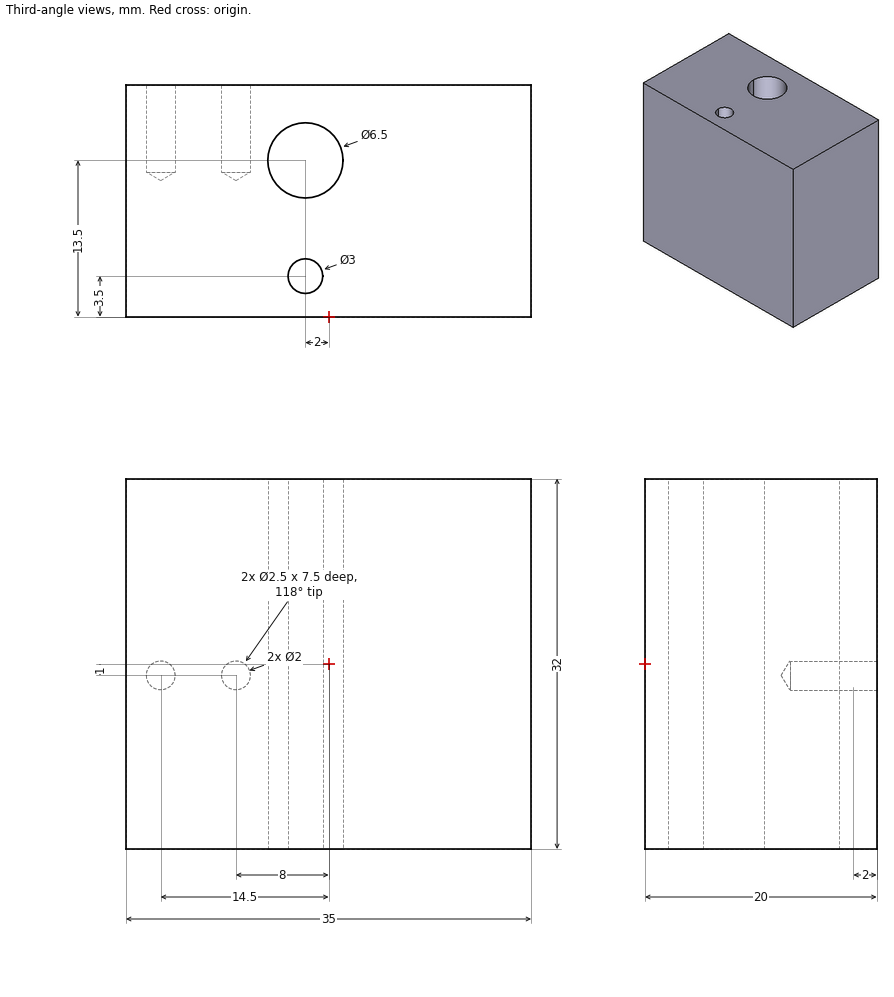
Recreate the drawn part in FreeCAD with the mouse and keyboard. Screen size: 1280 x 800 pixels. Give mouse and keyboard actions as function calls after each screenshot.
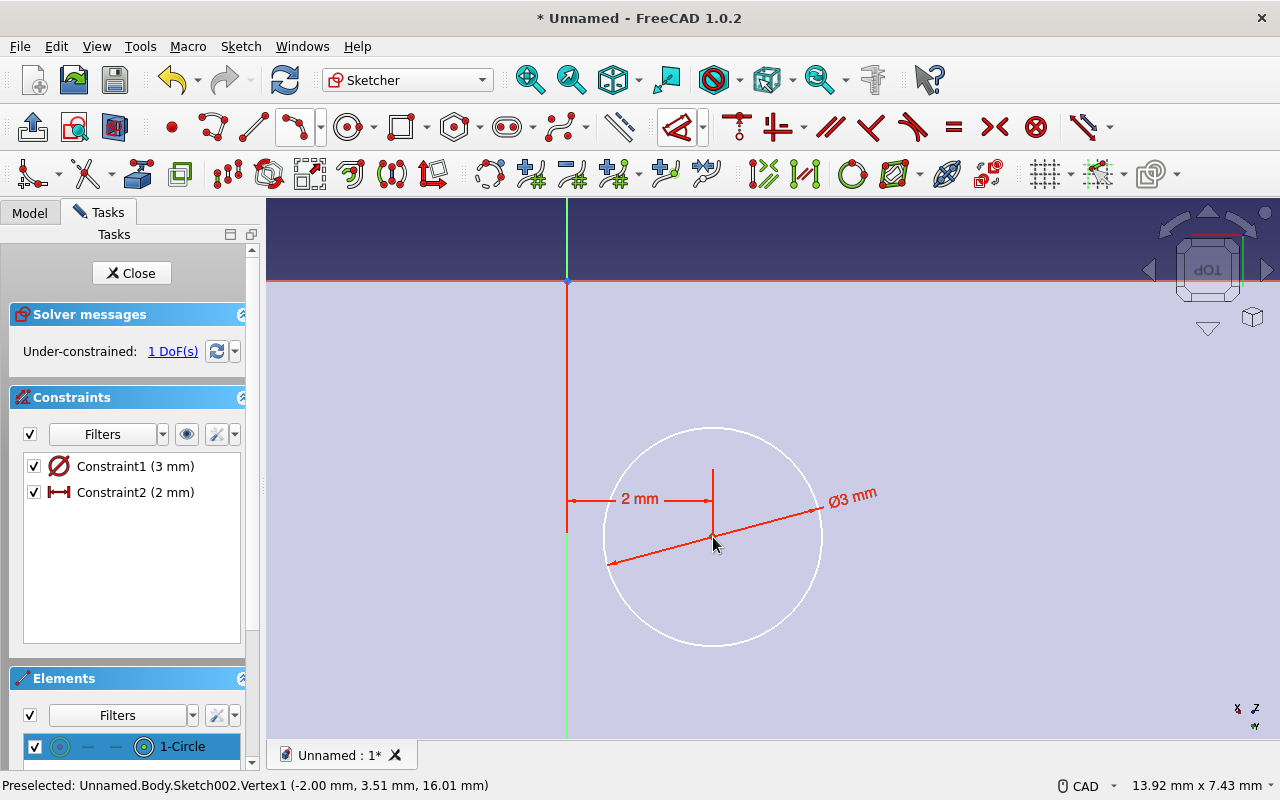
click(702, 128)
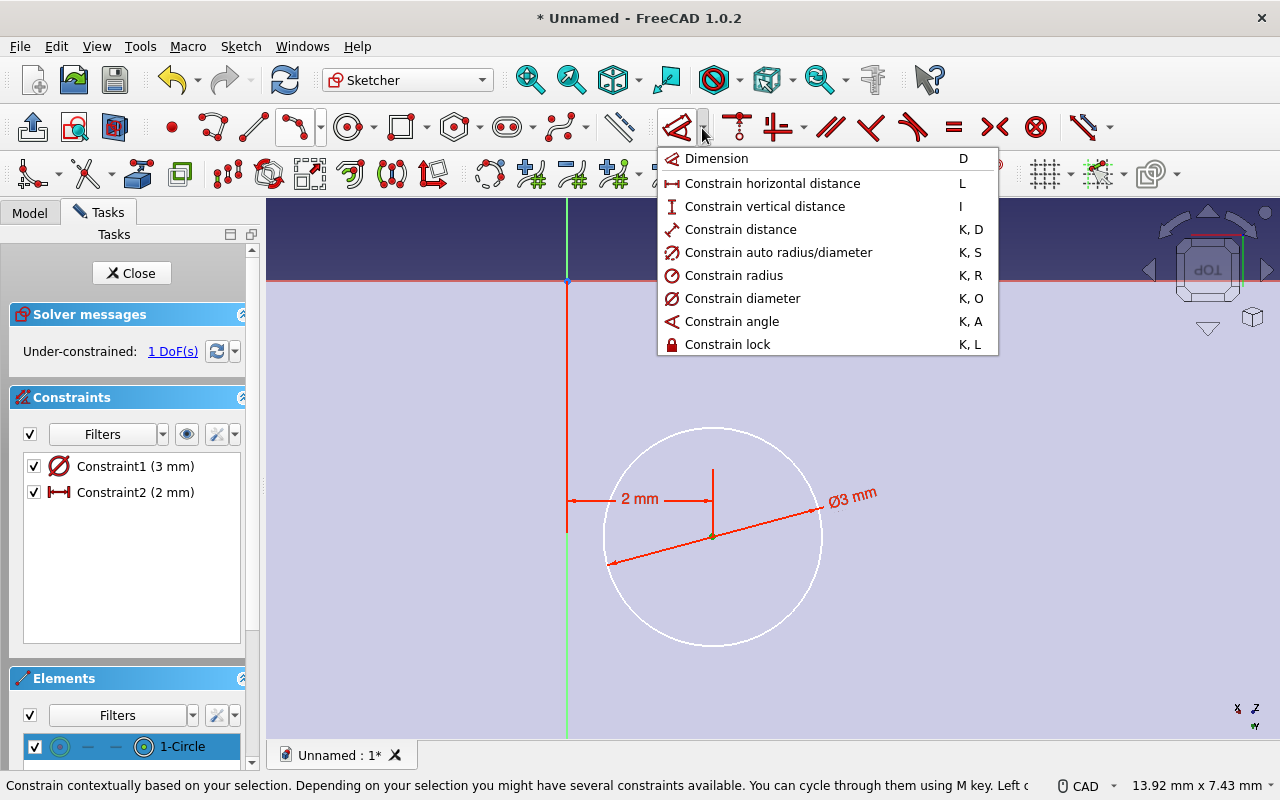
click(828, 206)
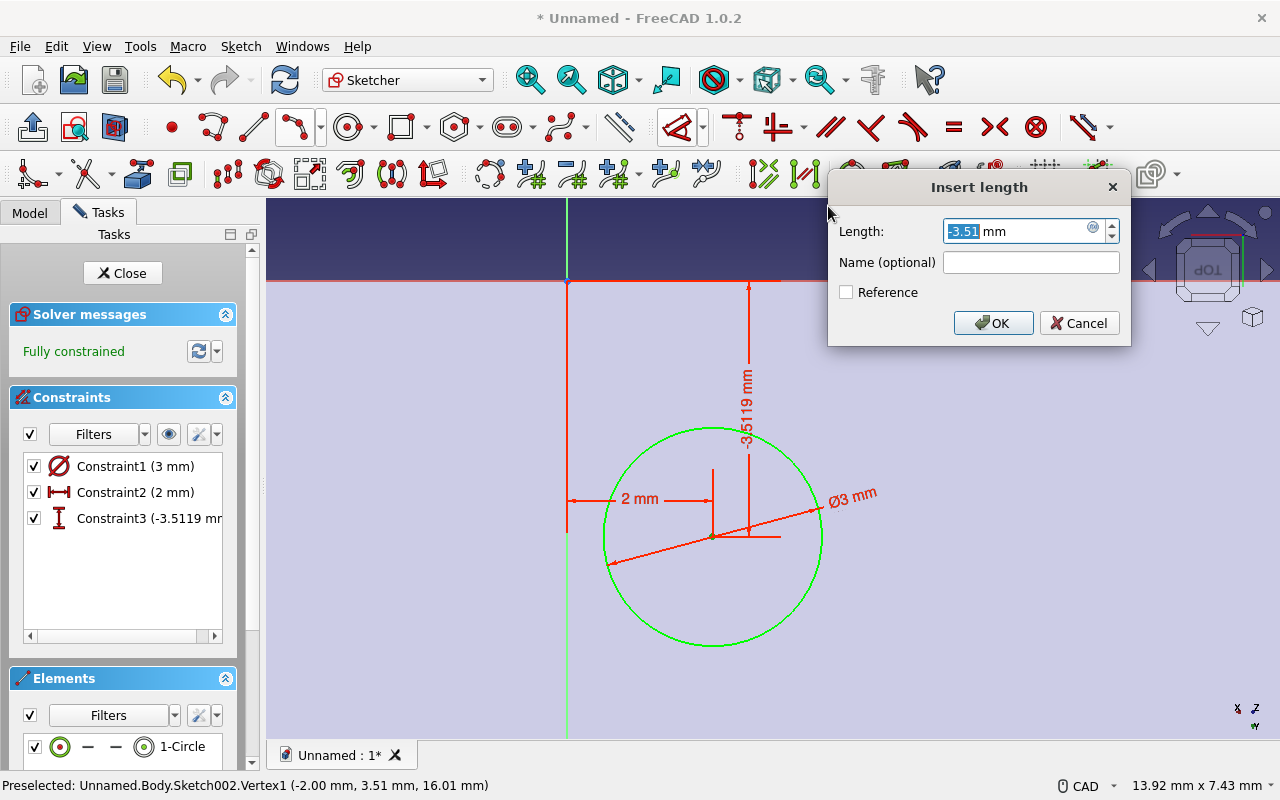
text(-3.5)
key(Return)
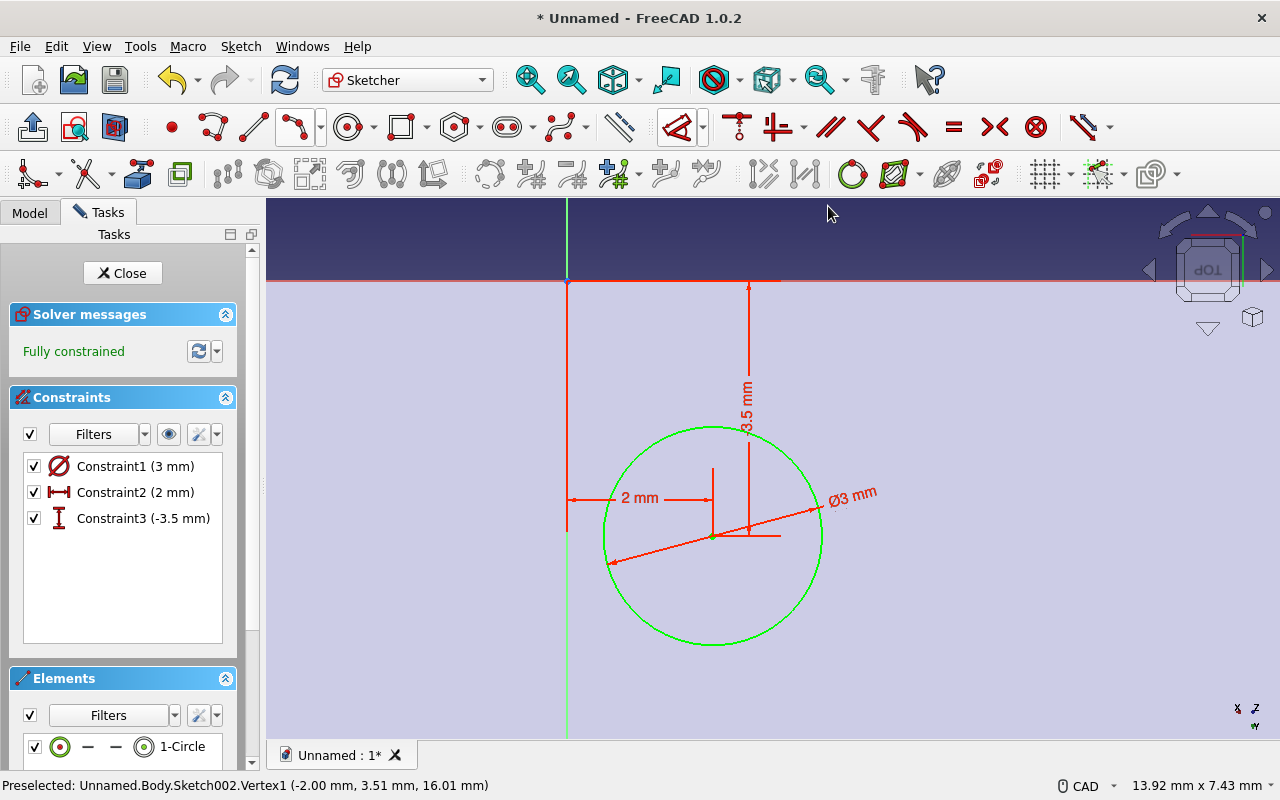
click(123, 273)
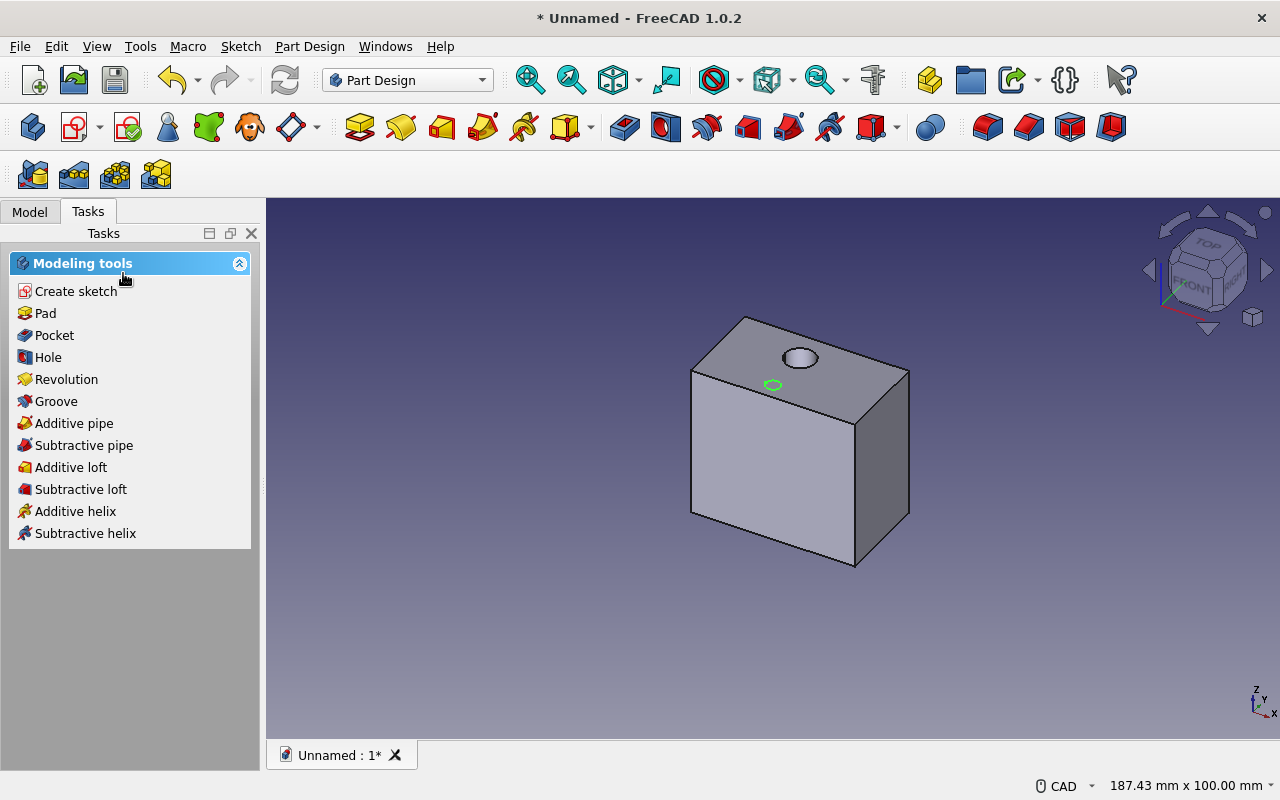
click(625, 128)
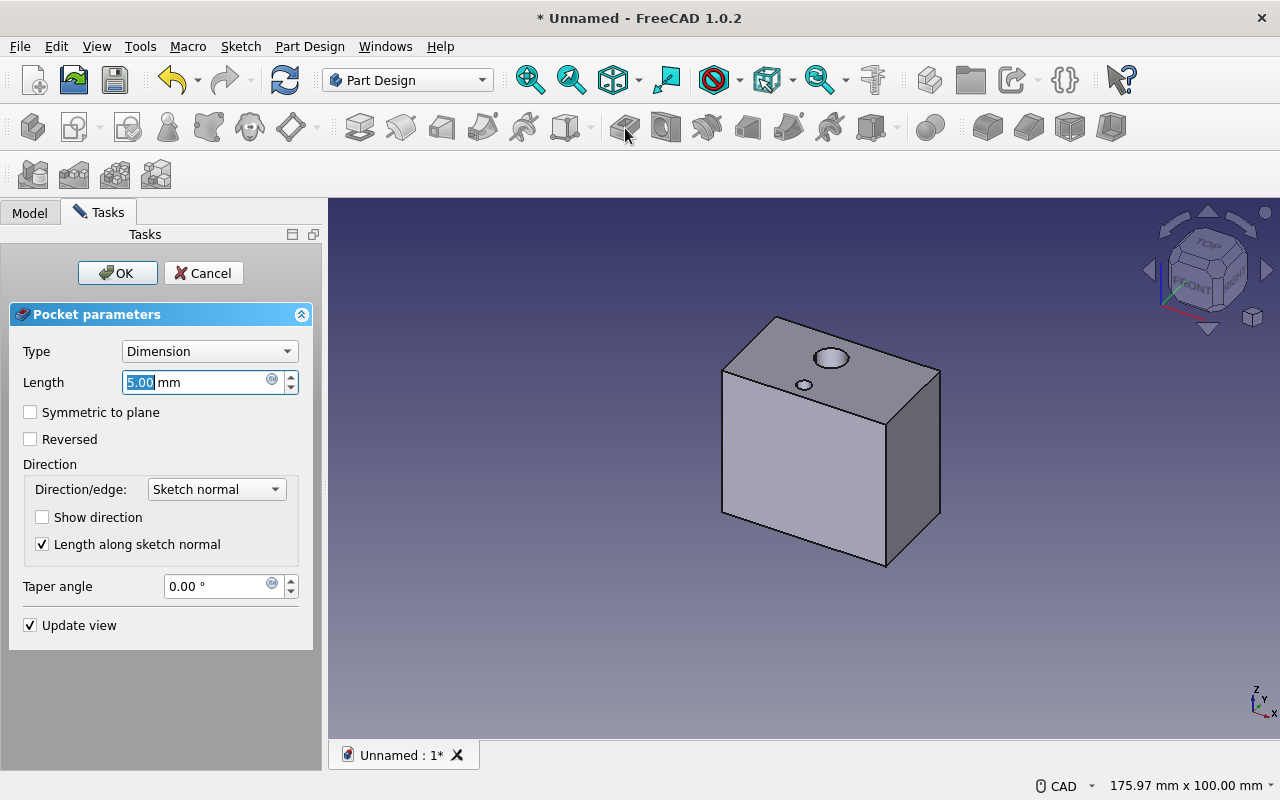
click(210, 352)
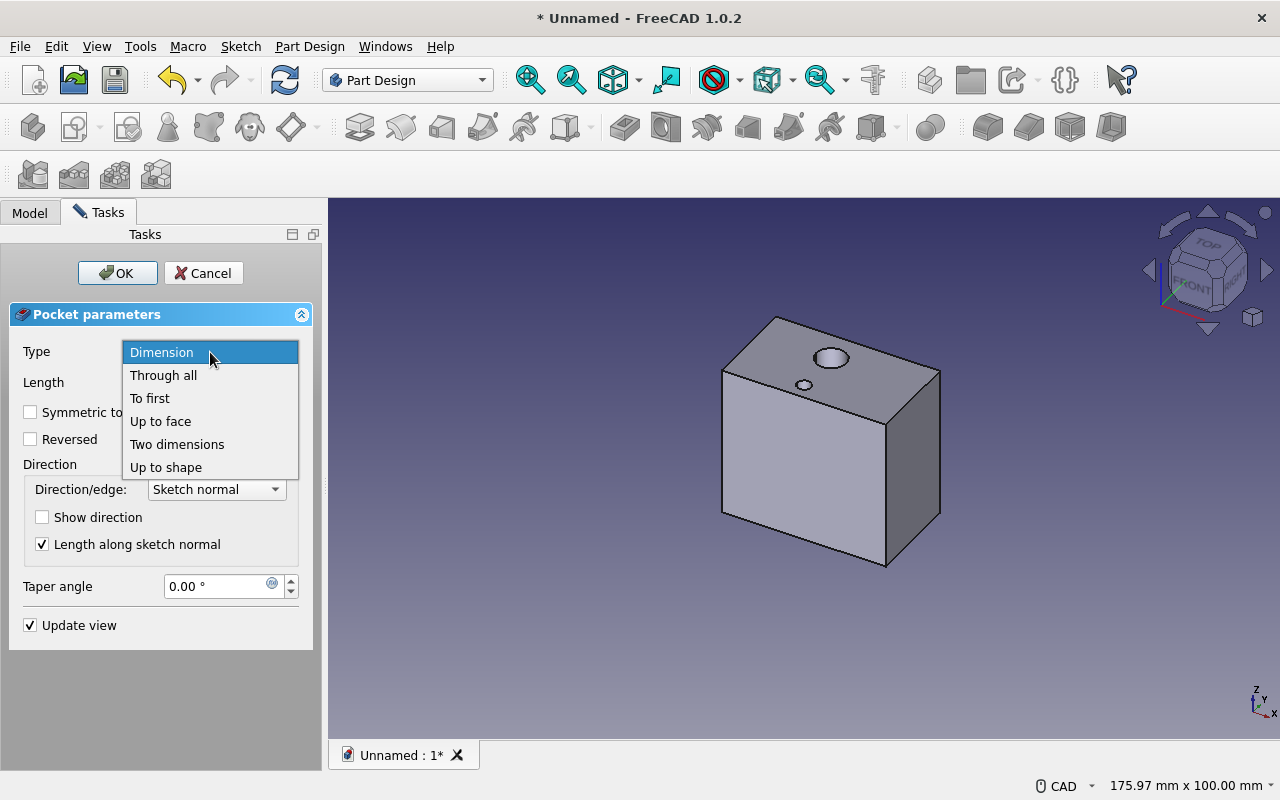
click(208, 398)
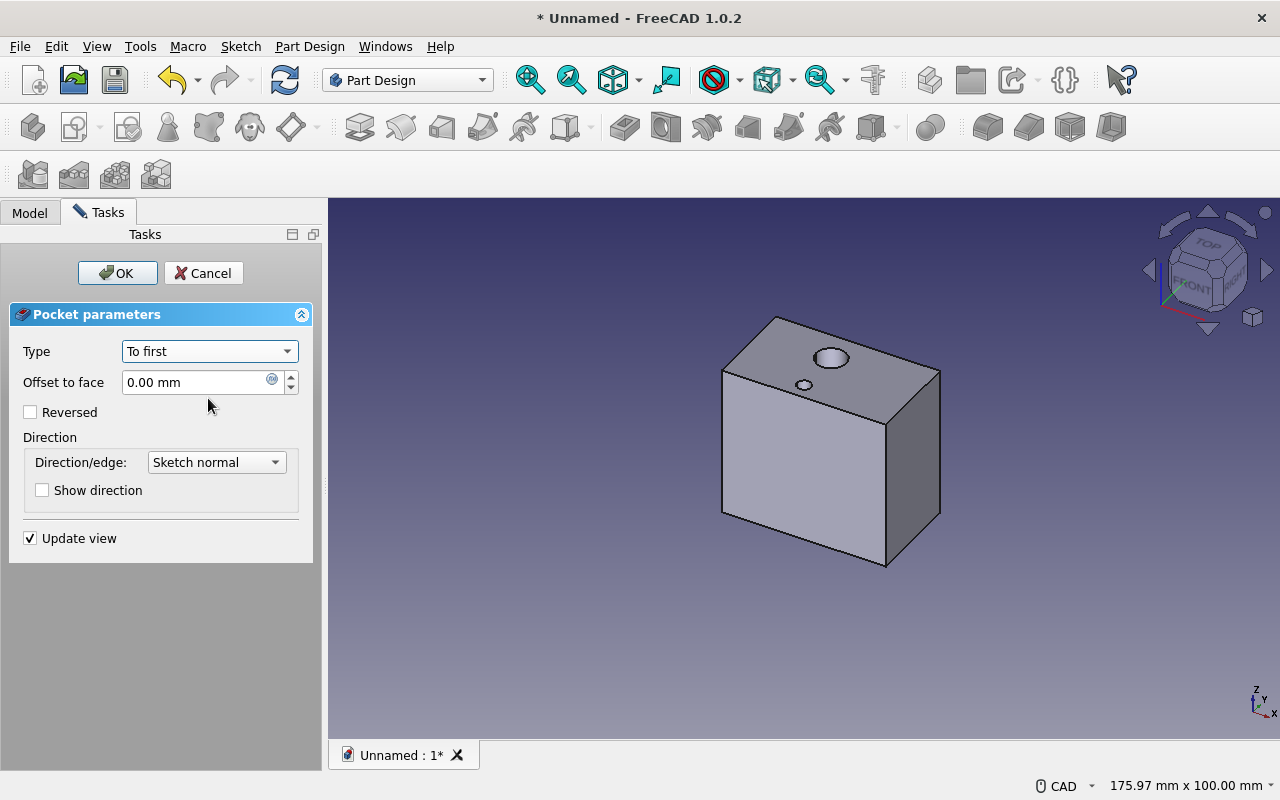
click(118, 273)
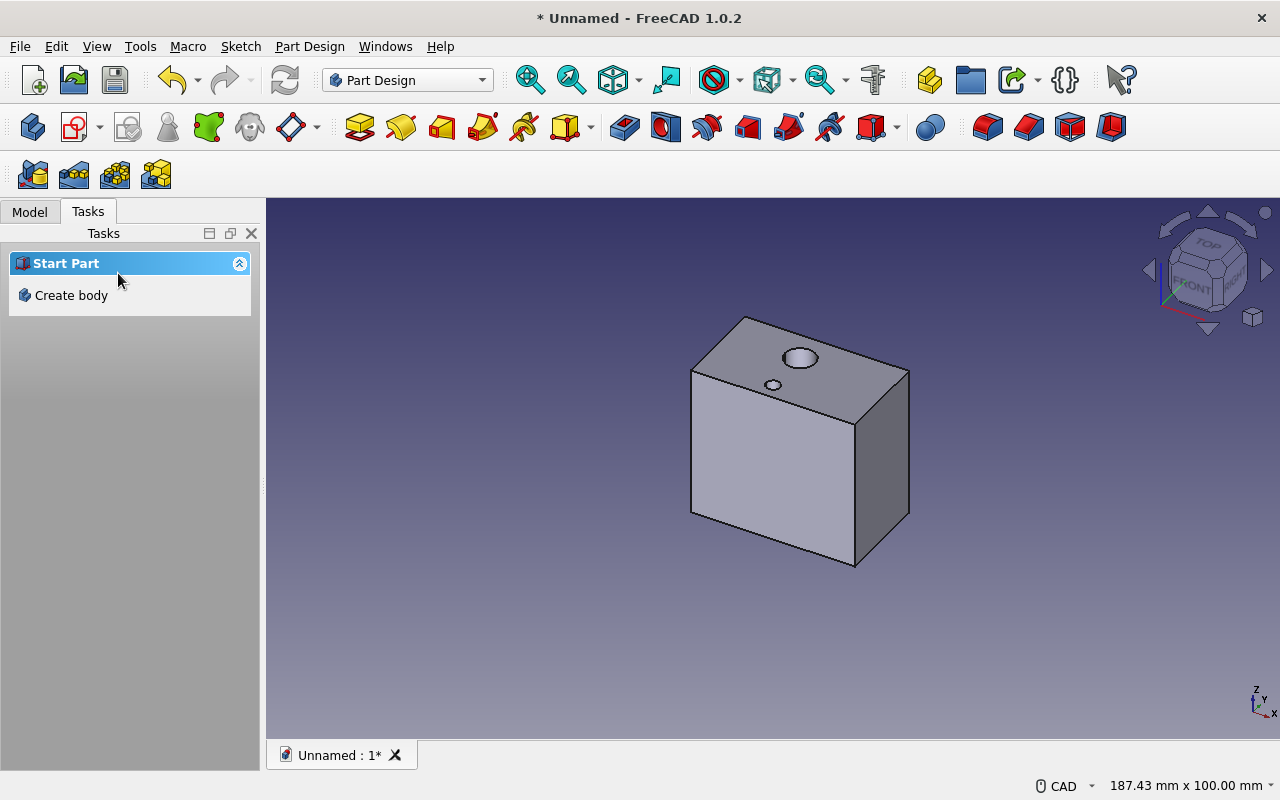
key(4)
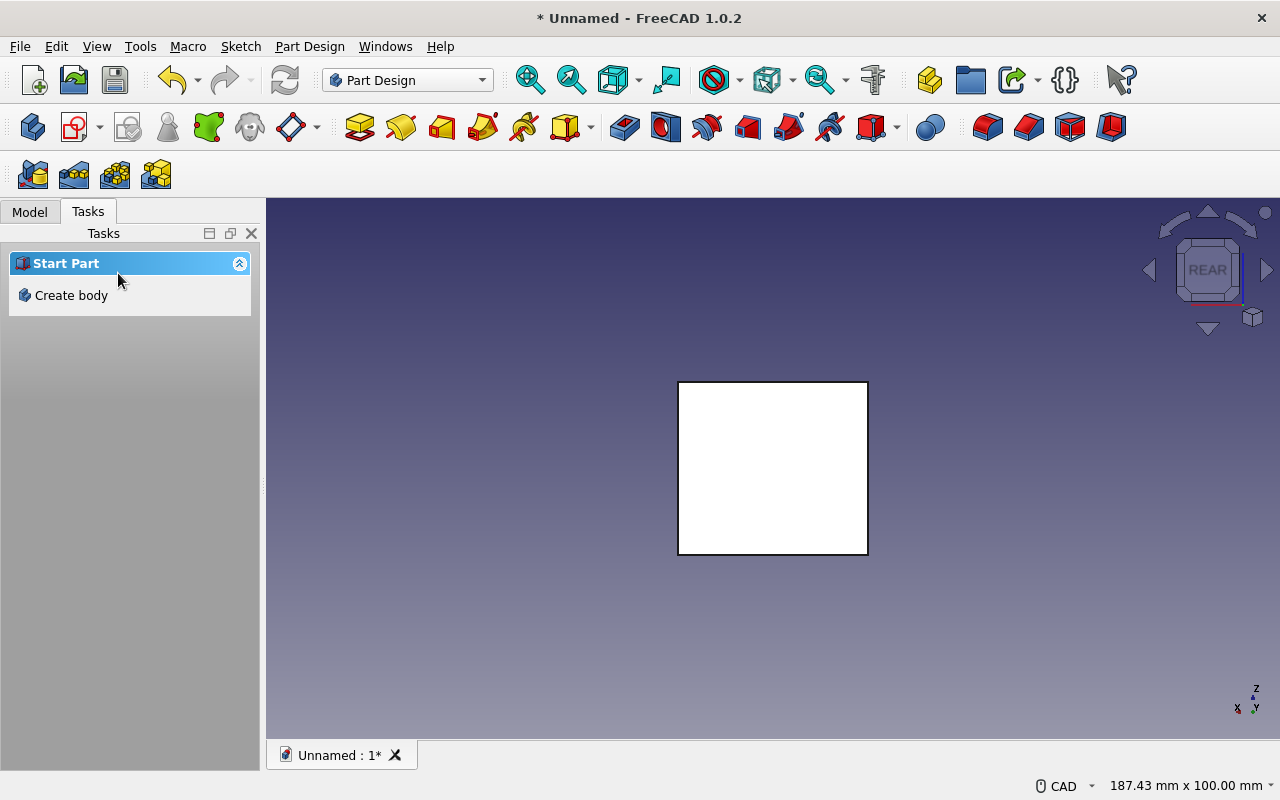
key(v)
key(f)